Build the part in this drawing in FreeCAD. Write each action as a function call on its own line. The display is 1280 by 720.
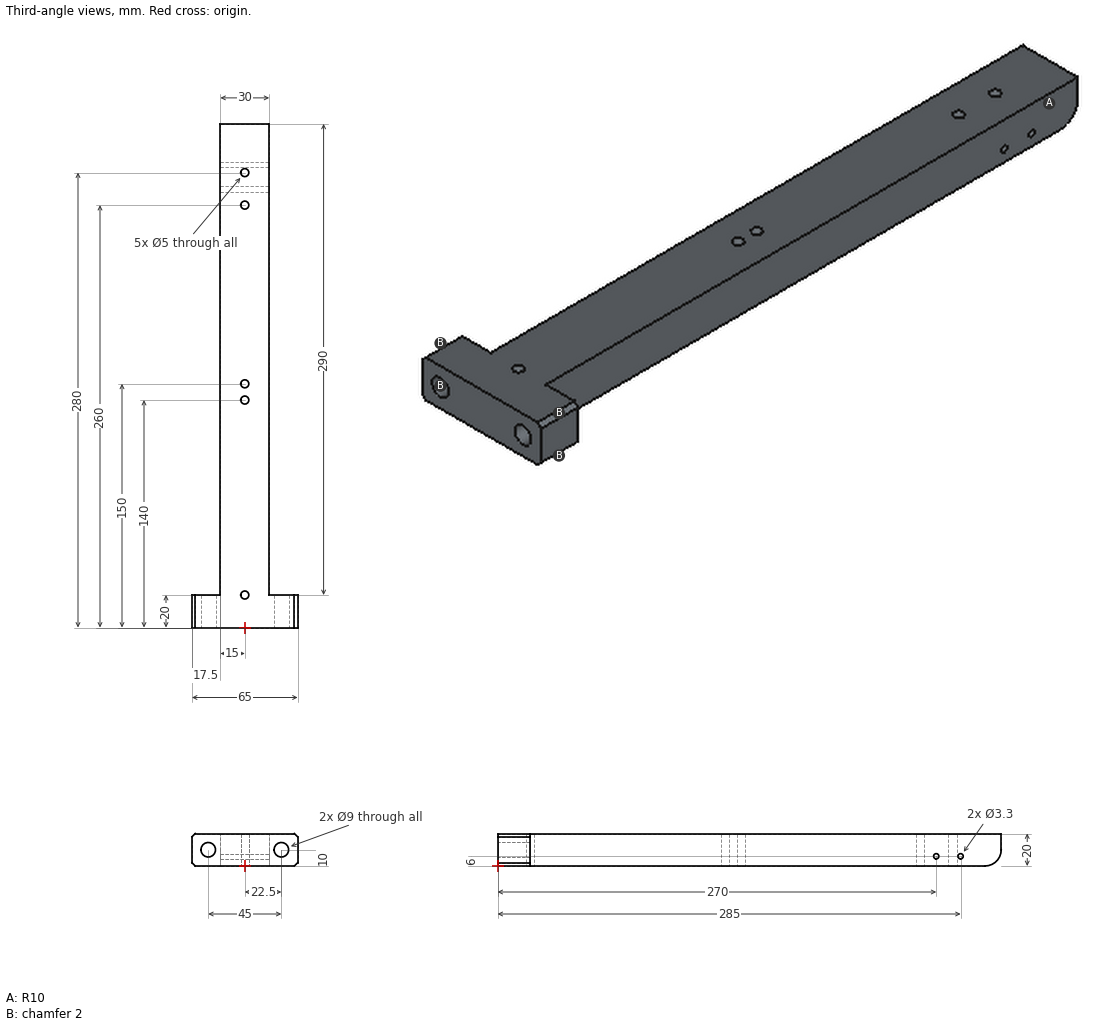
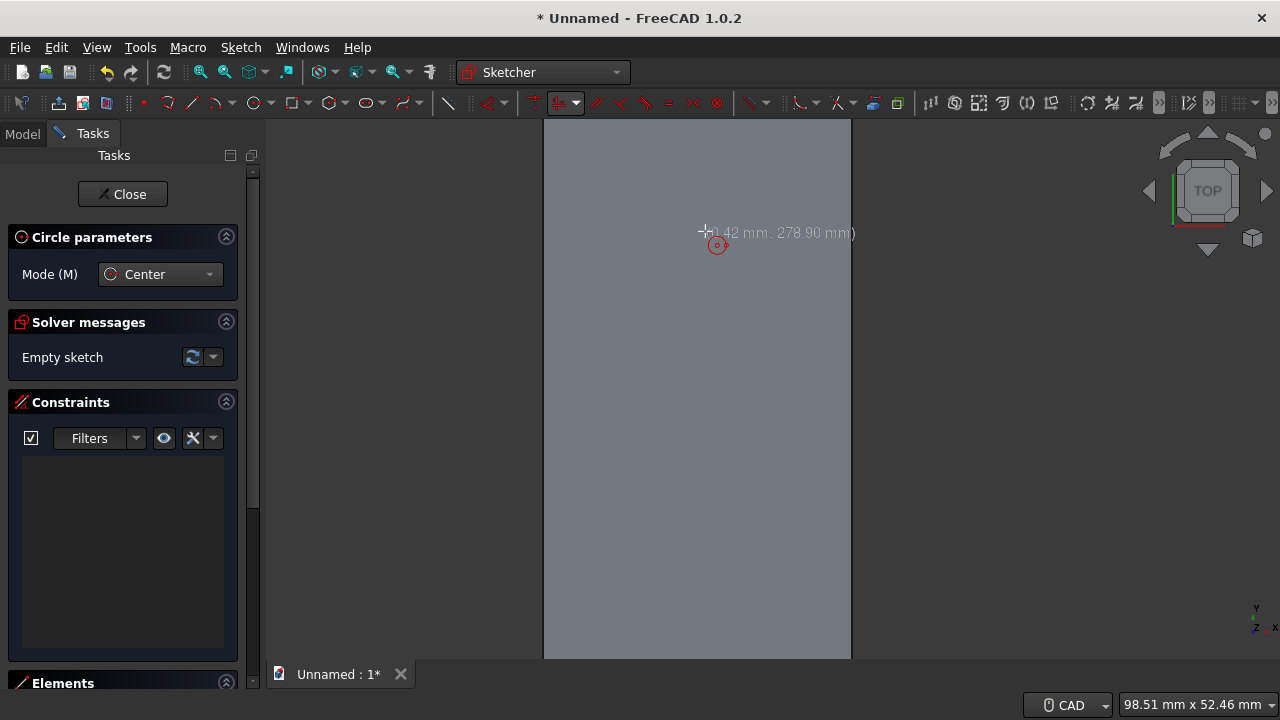
scroll(705, 231, down, 11)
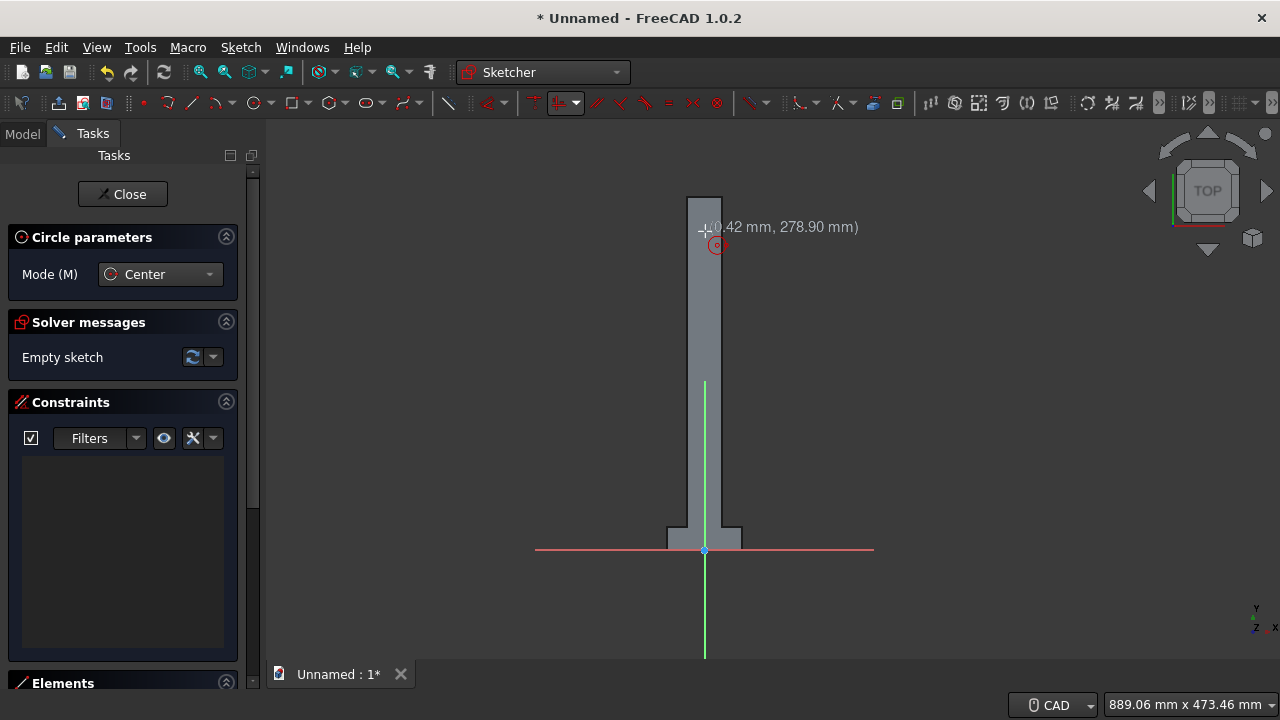
click(705, 231)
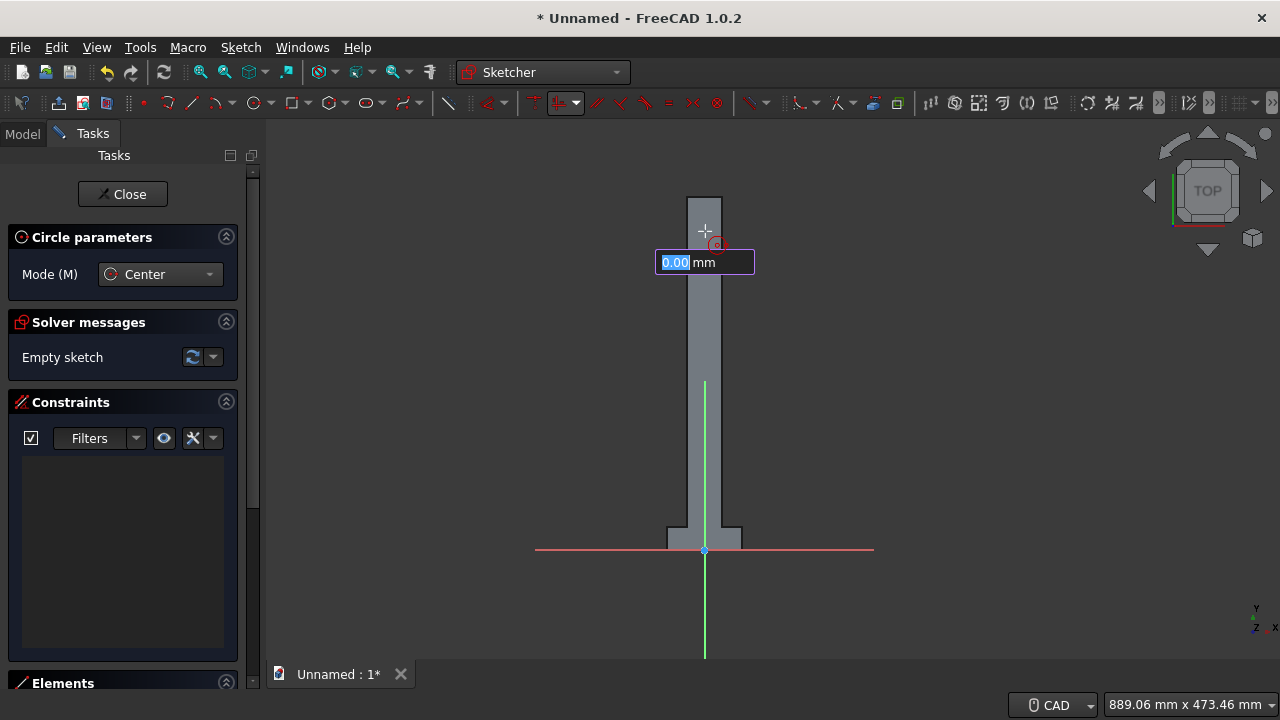
scroll(707, 230, up, 9)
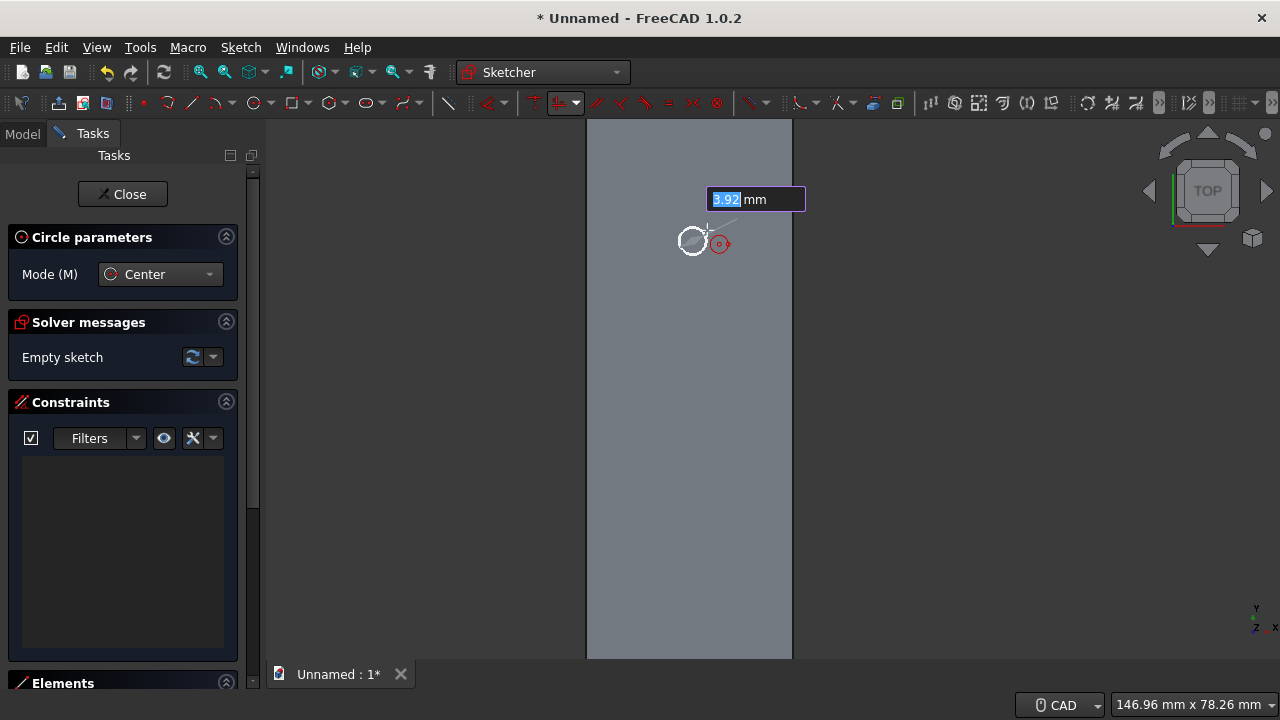
click(706, 228)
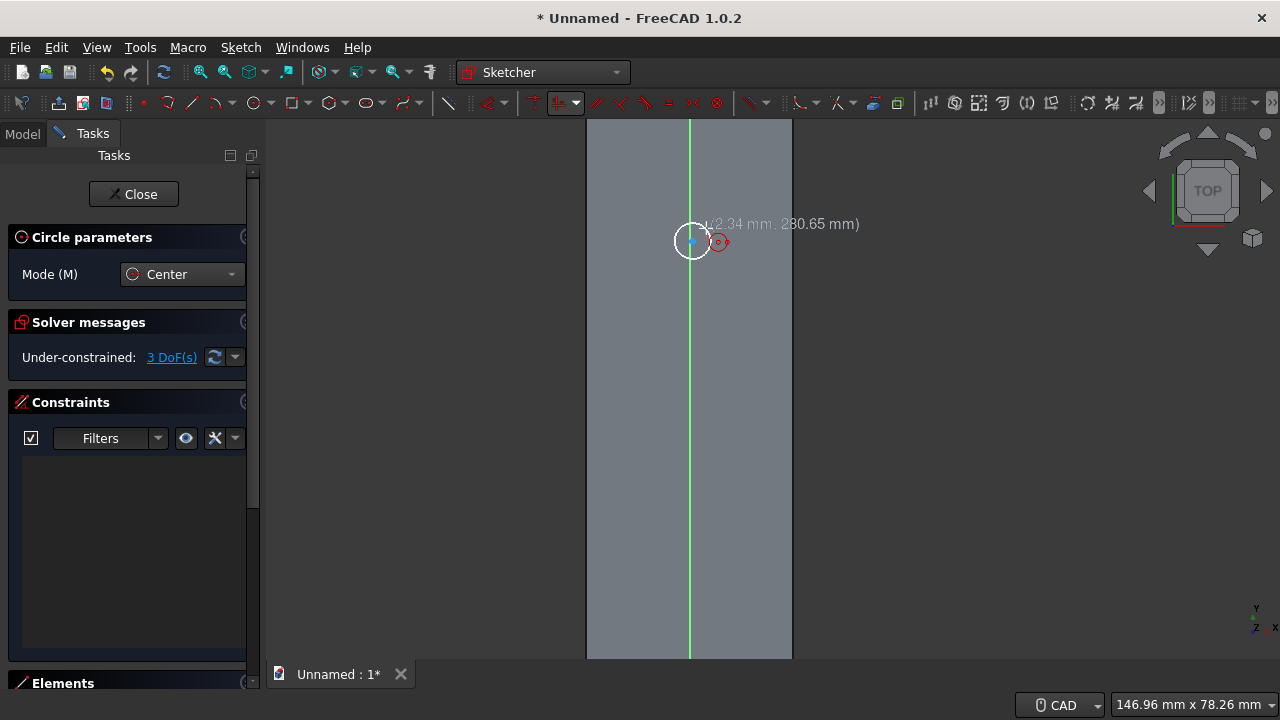
scroll(707, 230, down, 9)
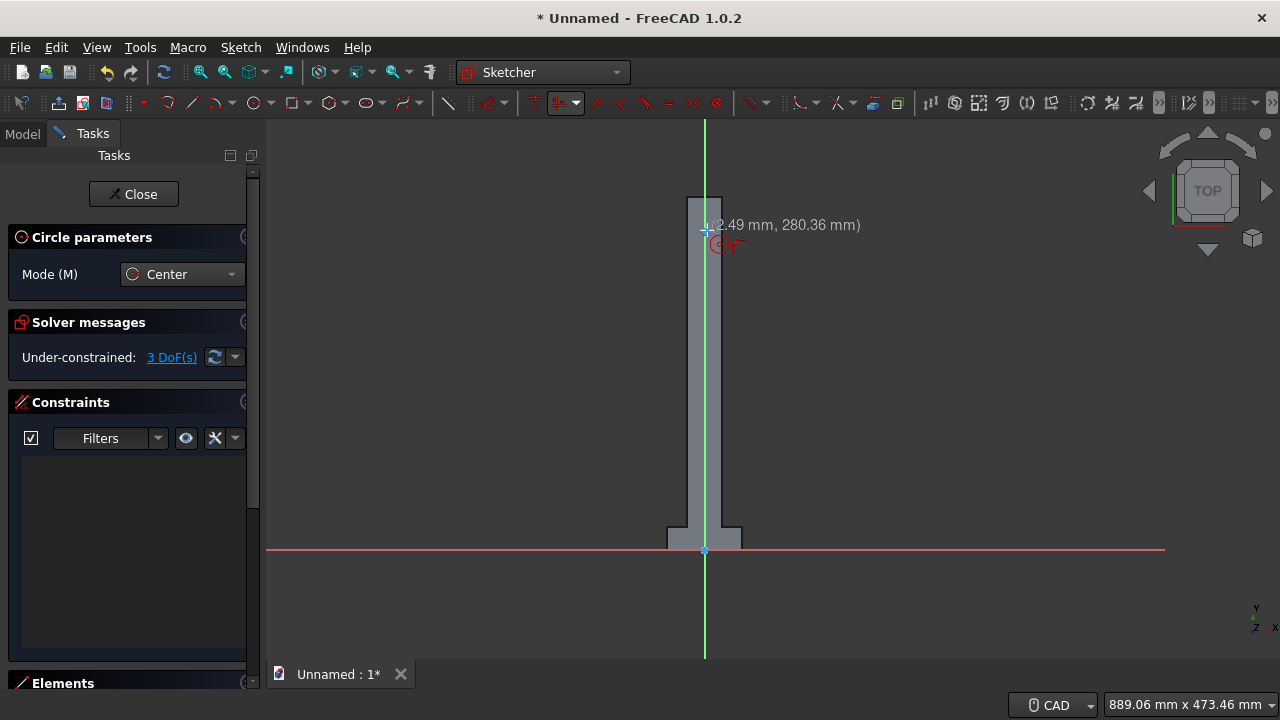
scroll(705, 379, up, 11)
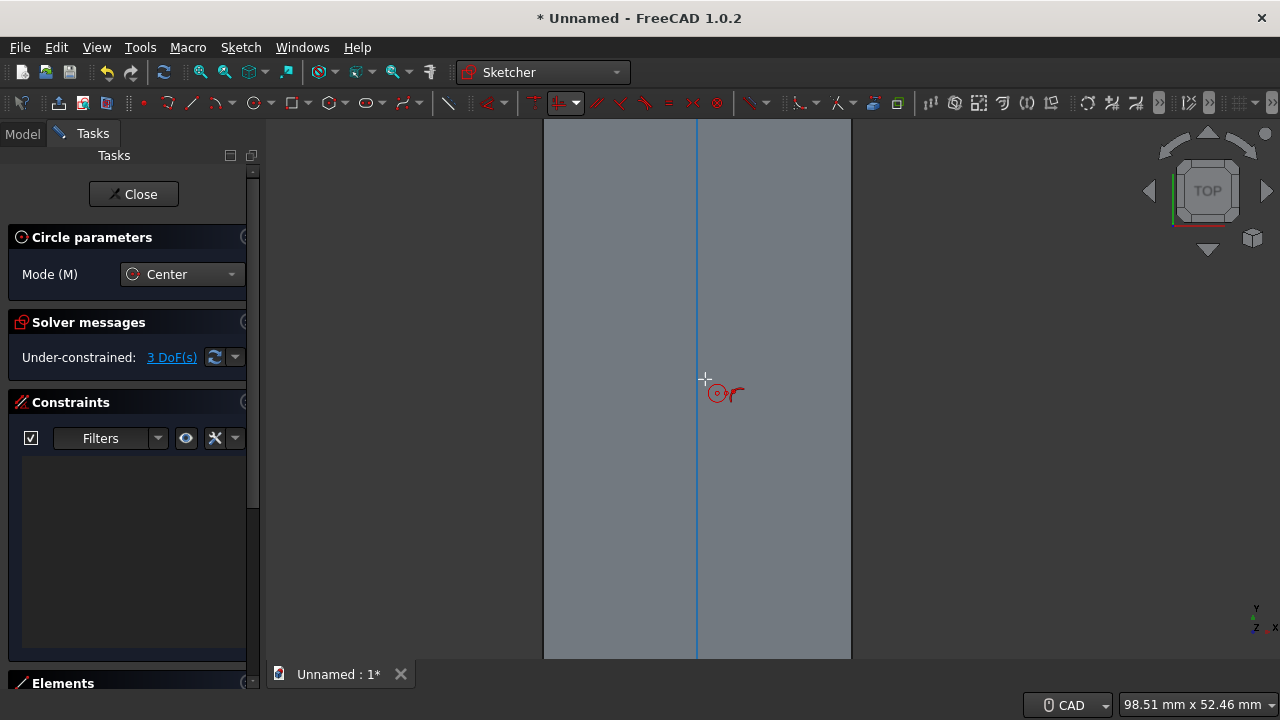
scroll(705, 379, down, 11)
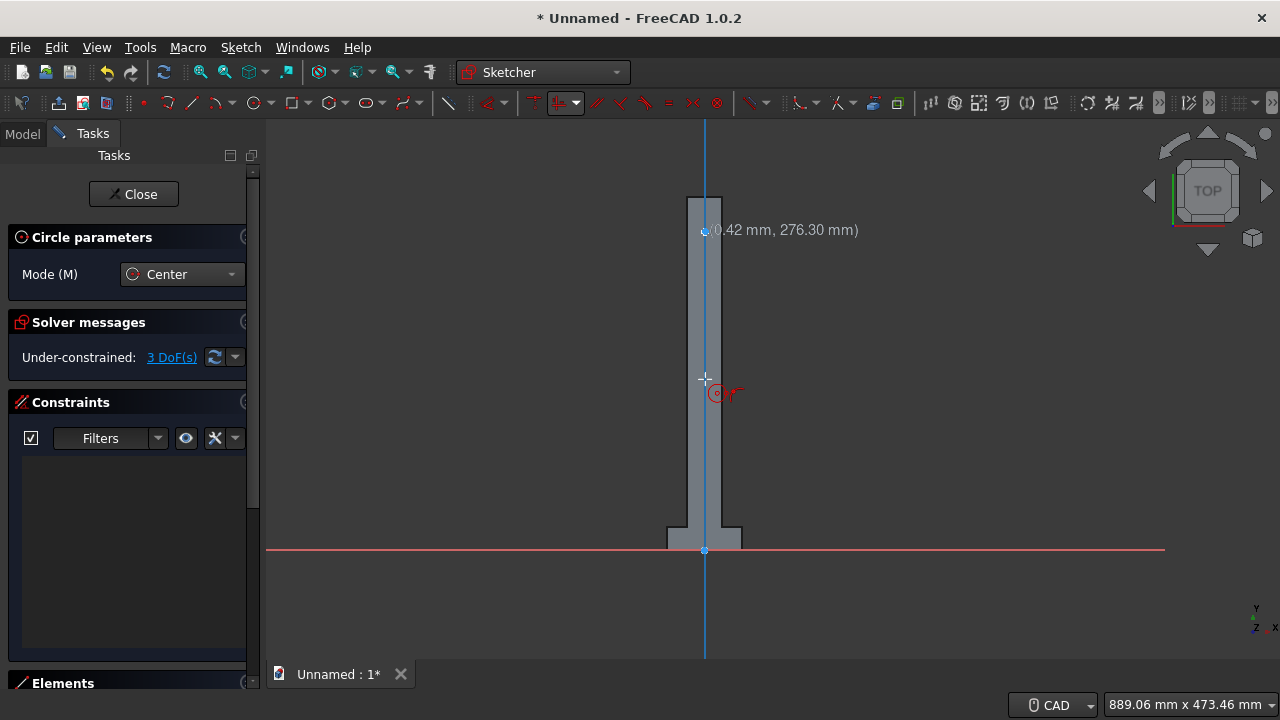
click(705, 379)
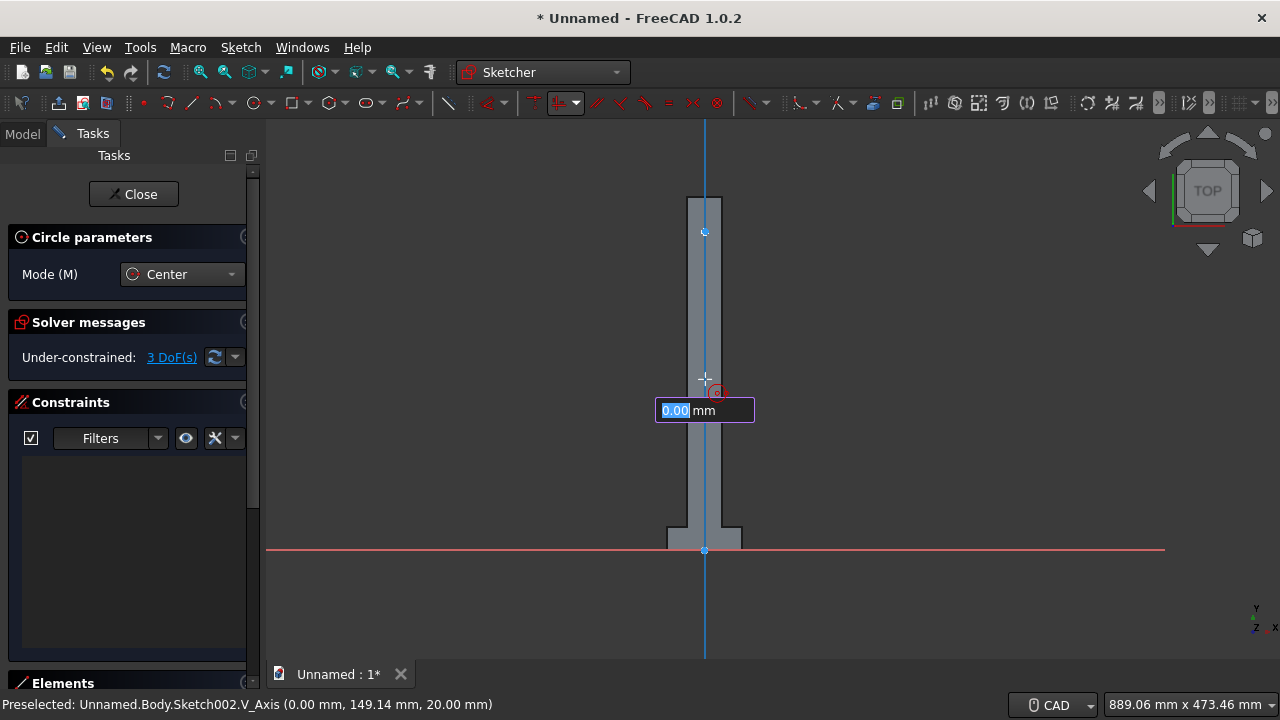
scroll(707, 378, up, 9)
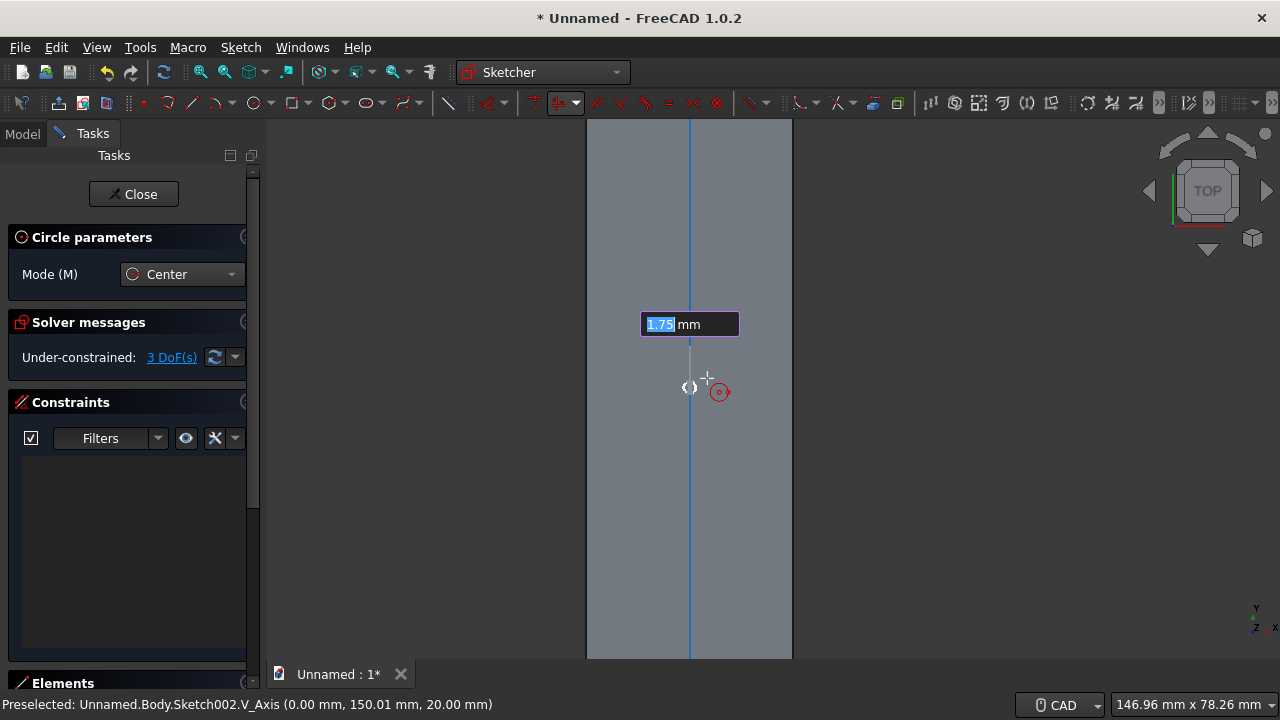
click(706, 376)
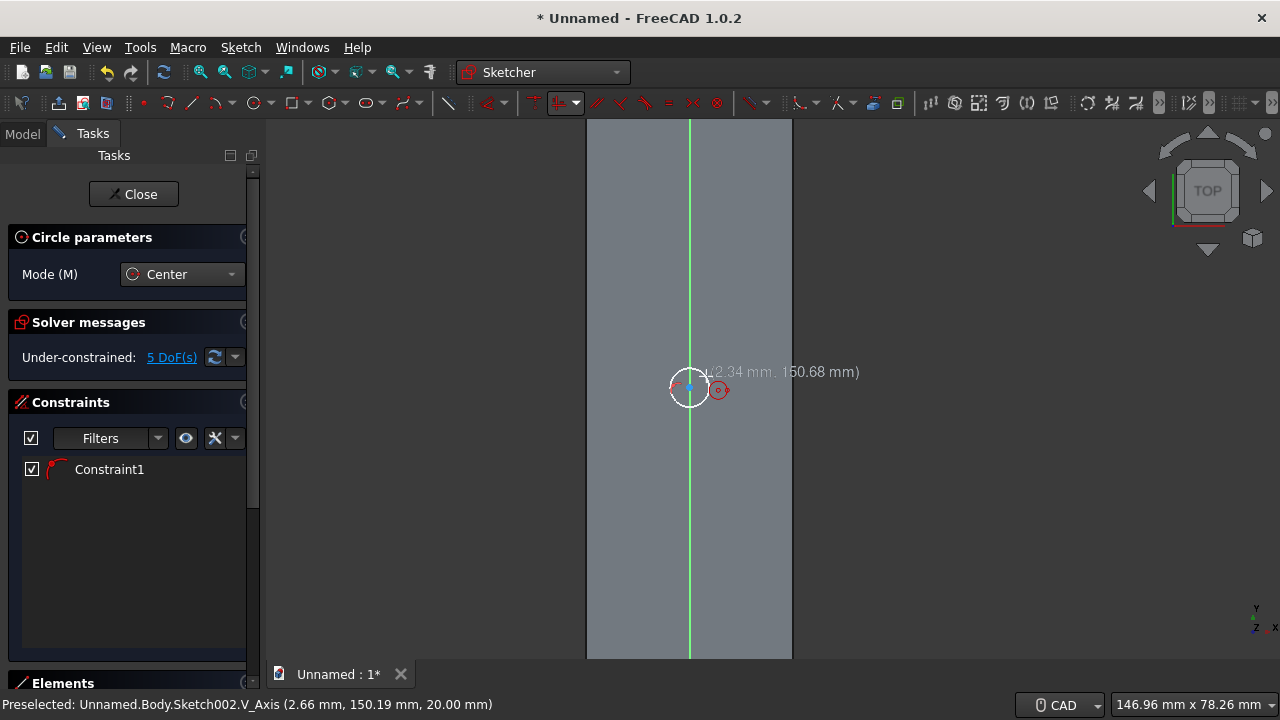
scroll(707, 378, down, 9)